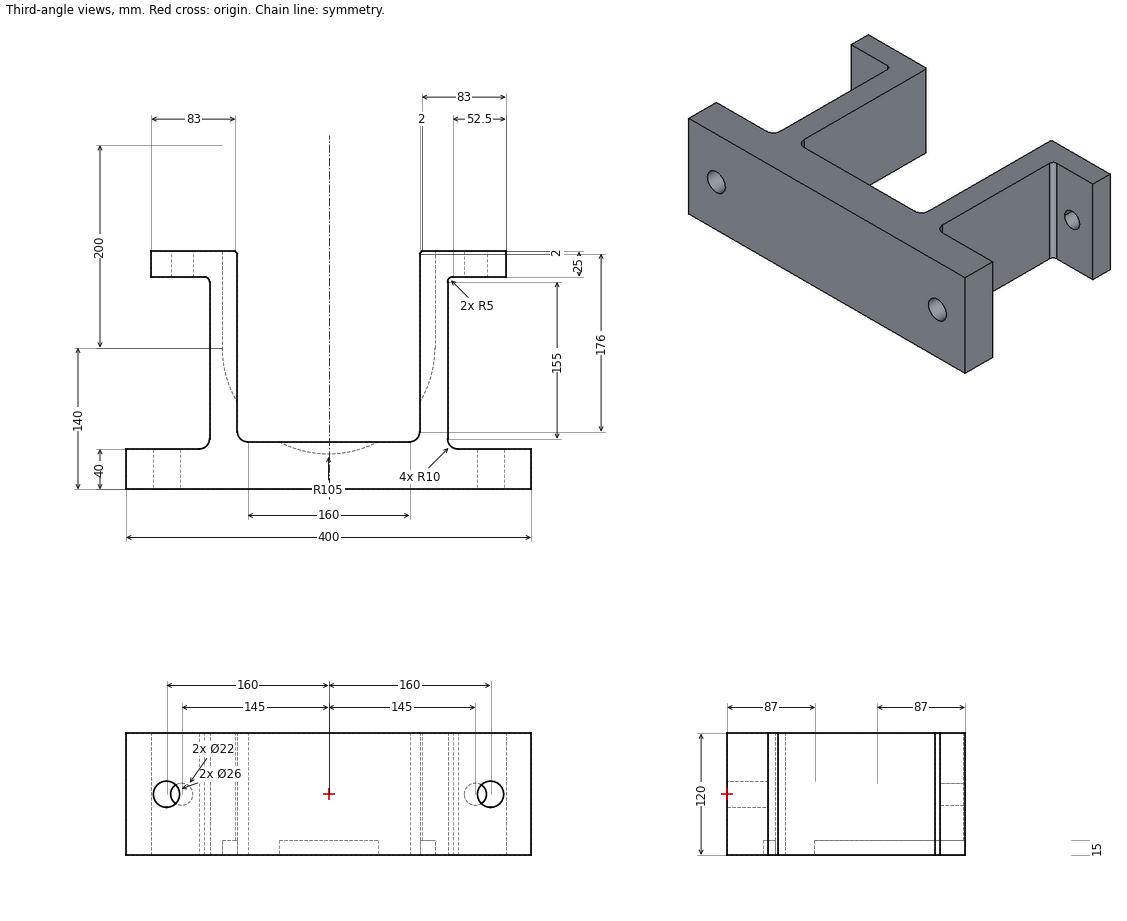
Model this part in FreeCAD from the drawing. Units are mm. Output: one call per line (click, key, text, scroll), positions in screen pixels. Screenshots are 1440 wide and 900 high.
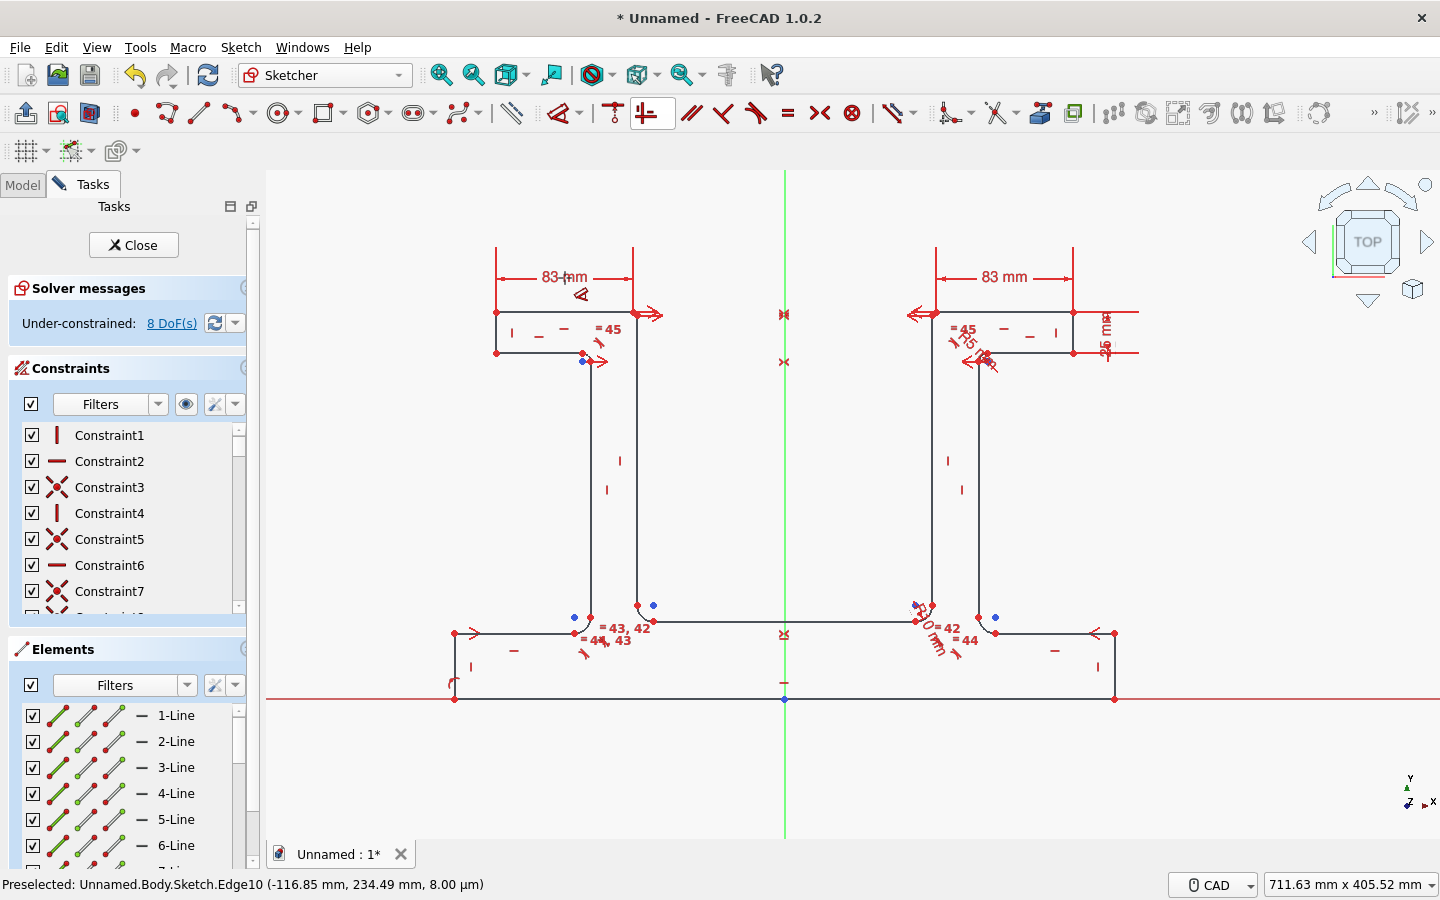
click(455, 653)
click(421, 666)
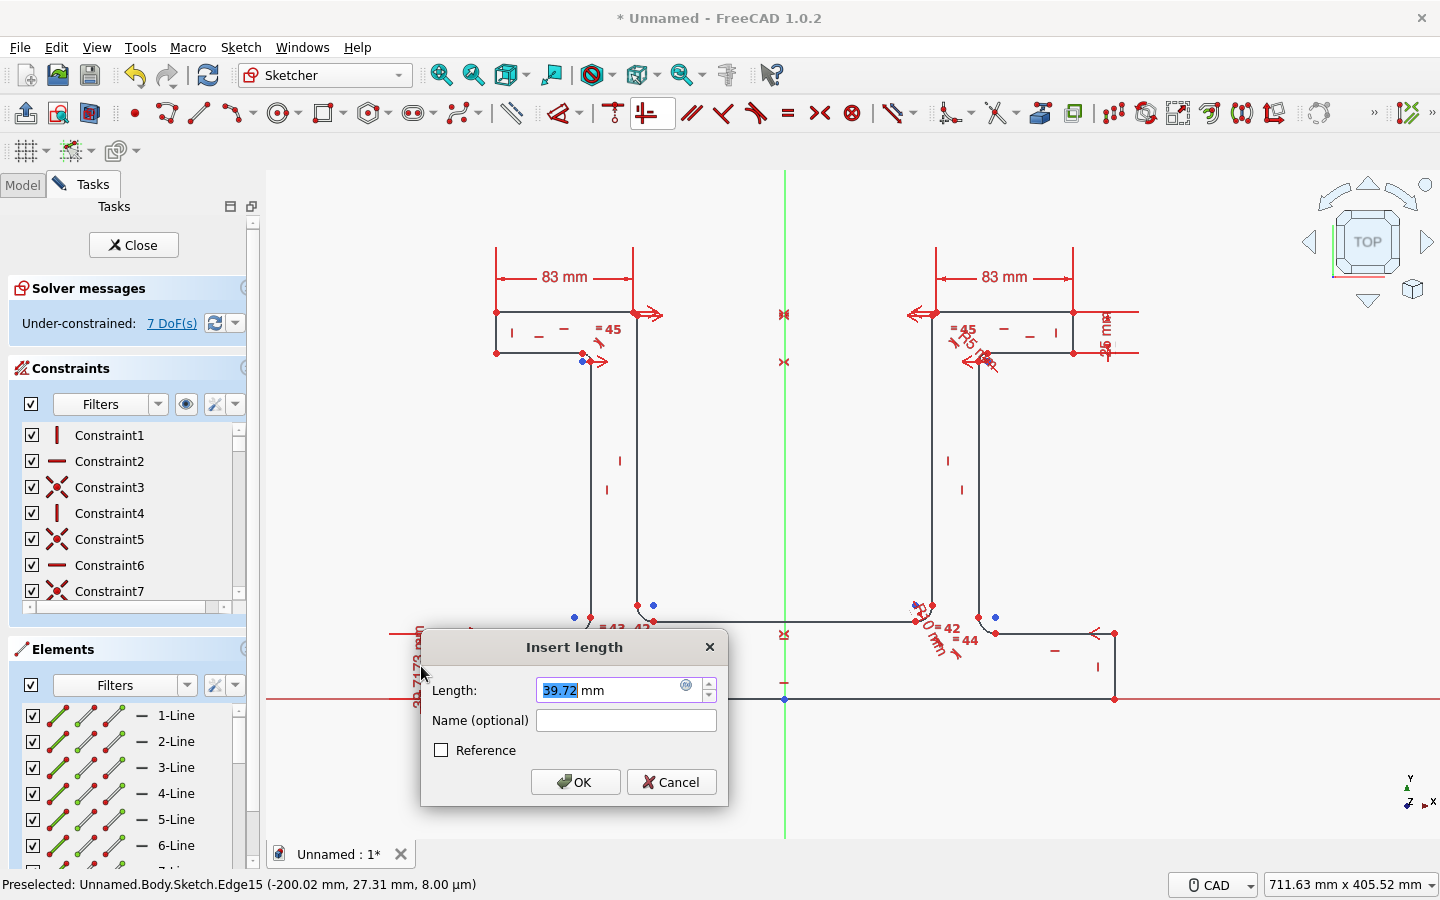
text(40)
key(Return)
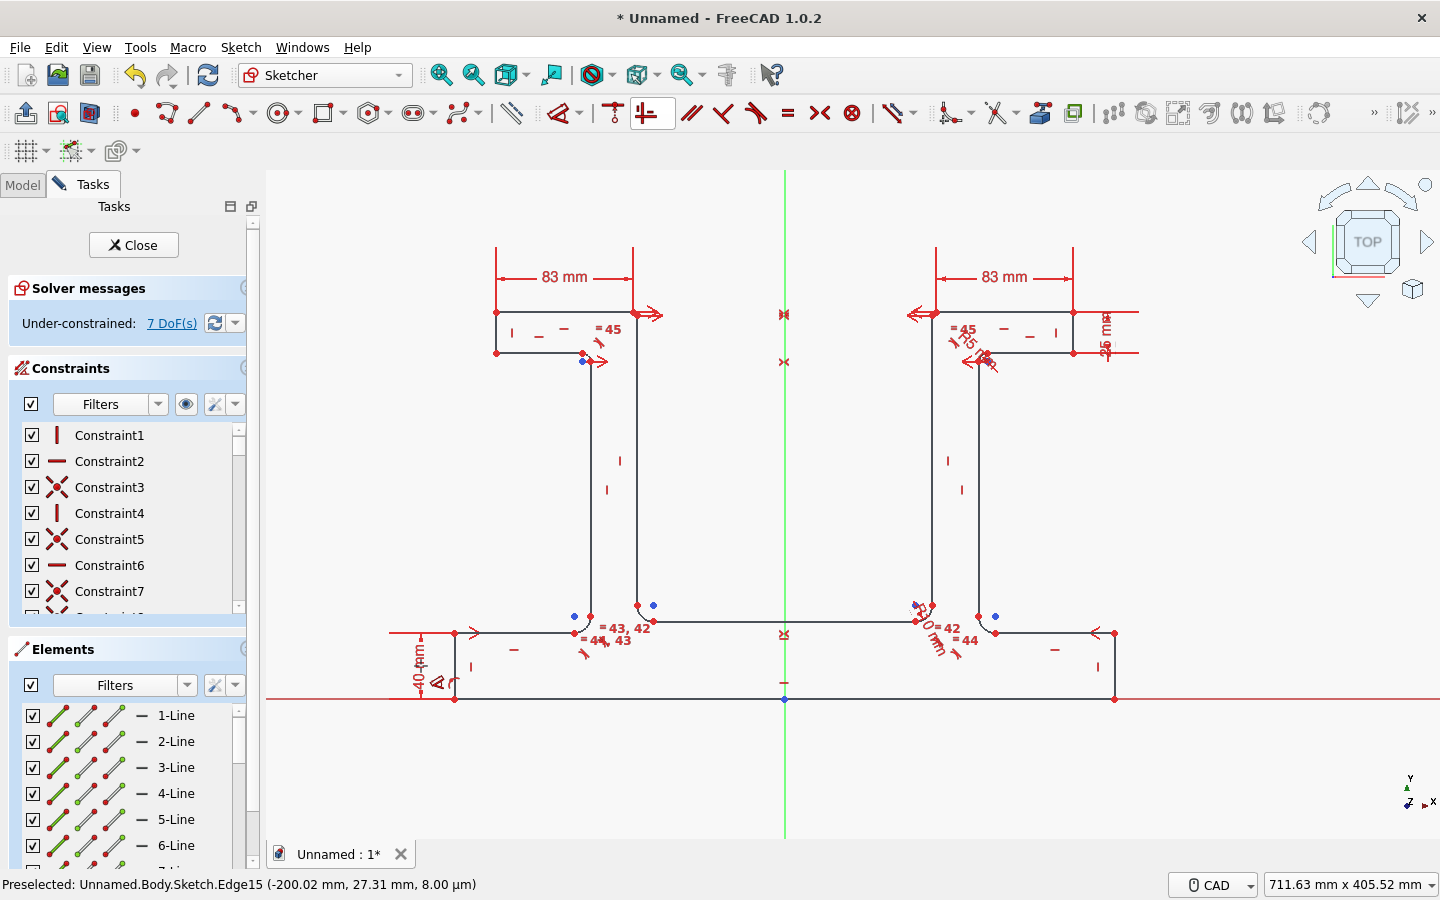
scroll(934, 314, up, 13)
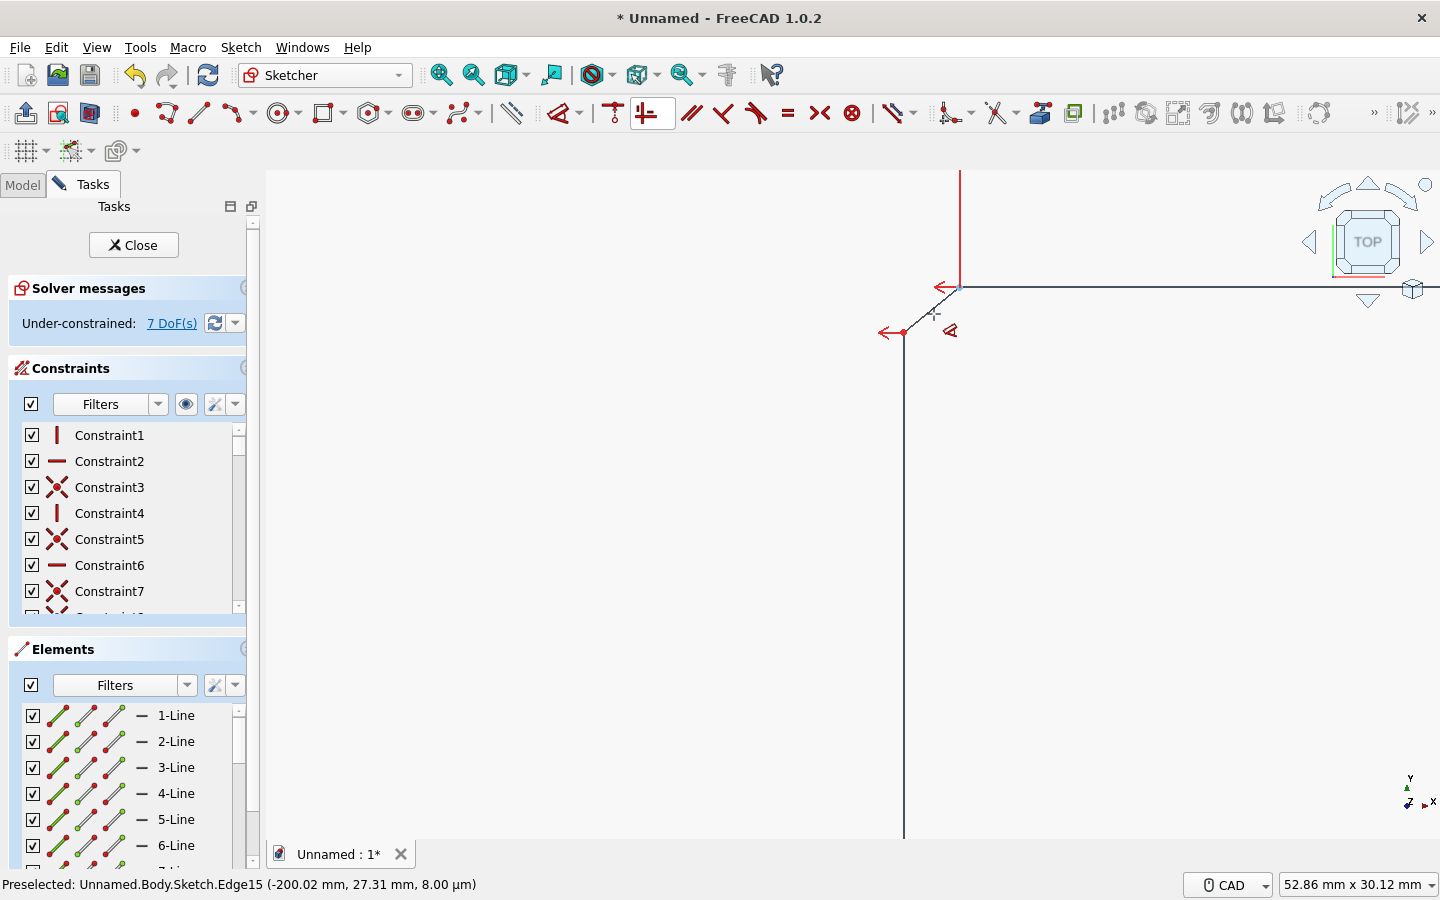
click(932, 310)
click(932, 253)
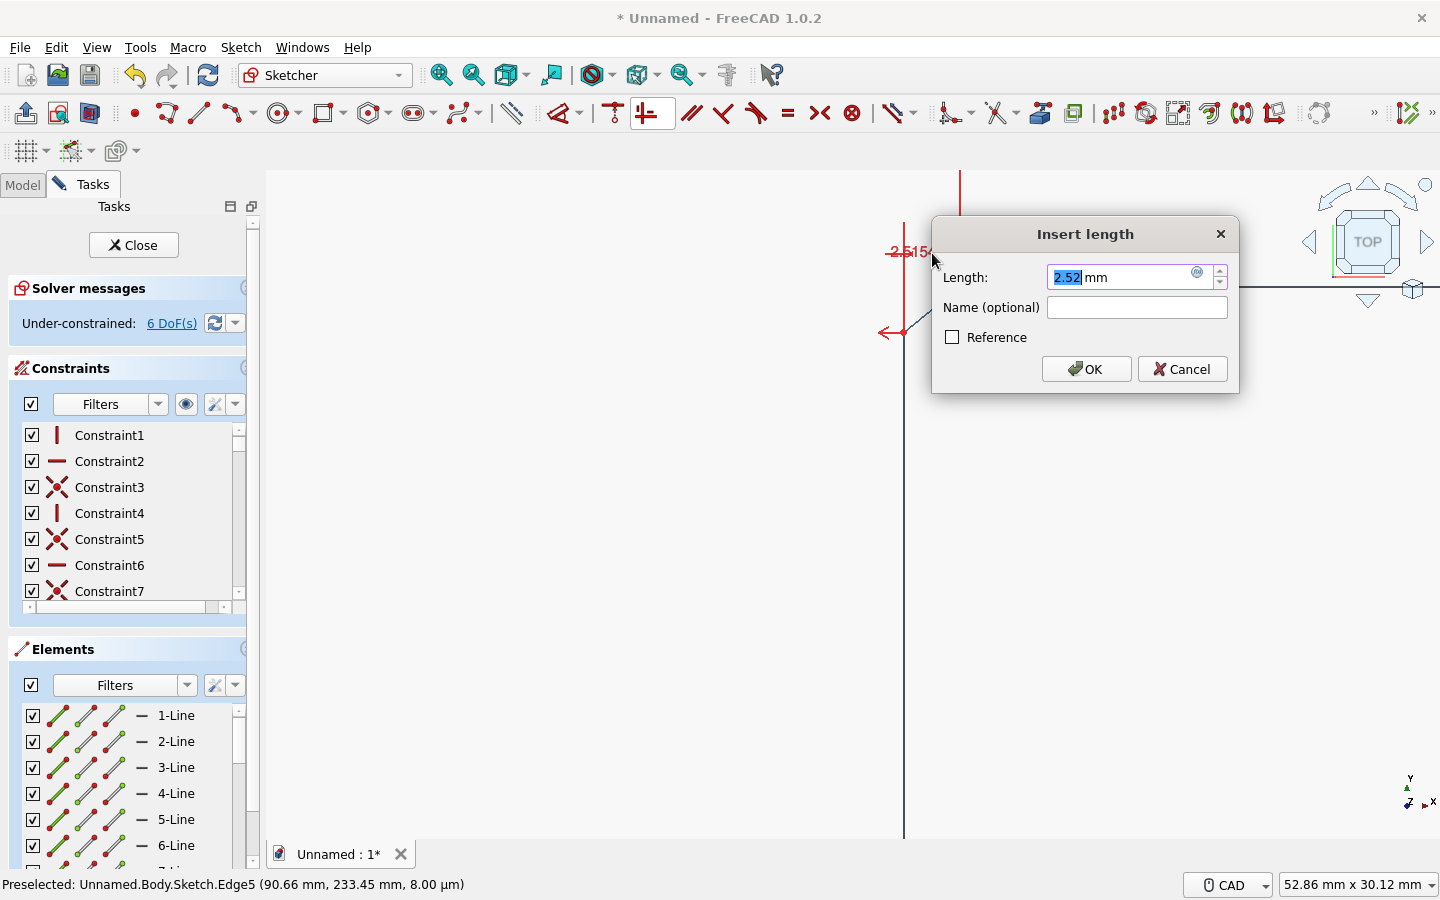
text(2)
key(Return)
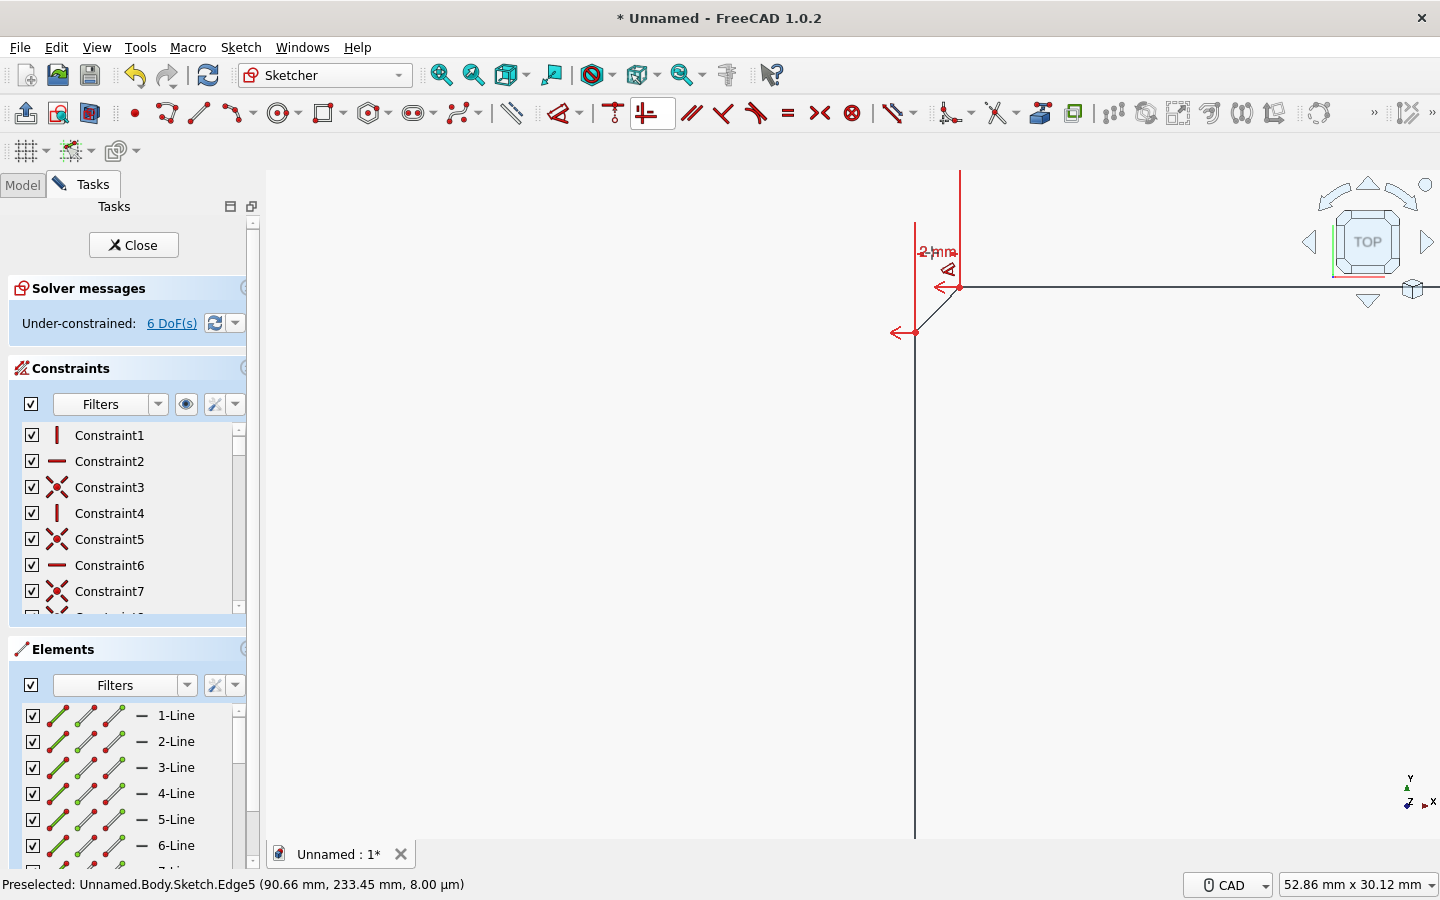
click(946, 301)
click(994, 310)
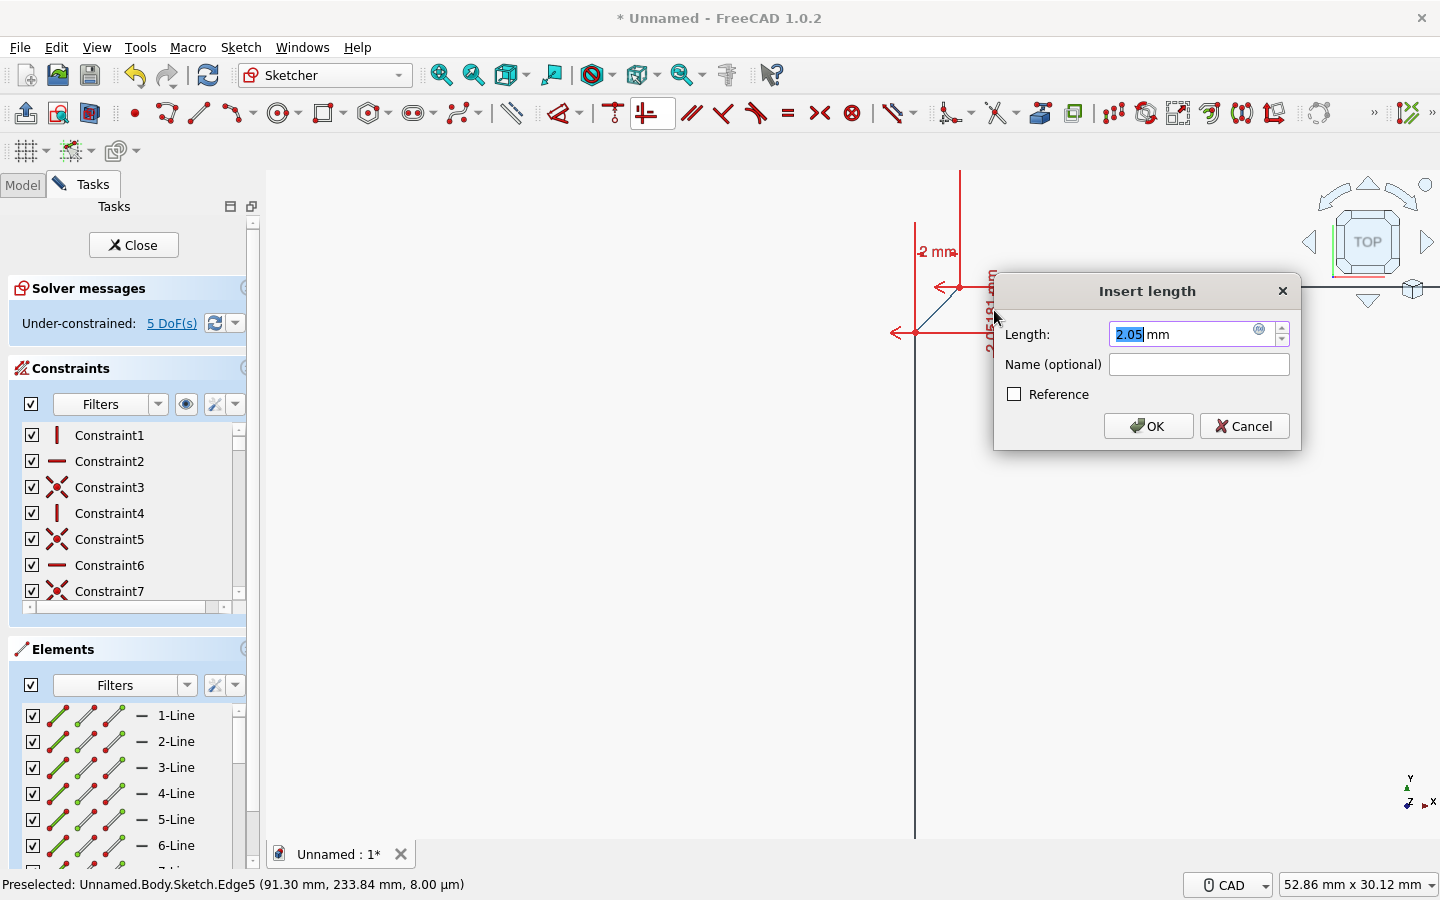
text(2)
key(Return)